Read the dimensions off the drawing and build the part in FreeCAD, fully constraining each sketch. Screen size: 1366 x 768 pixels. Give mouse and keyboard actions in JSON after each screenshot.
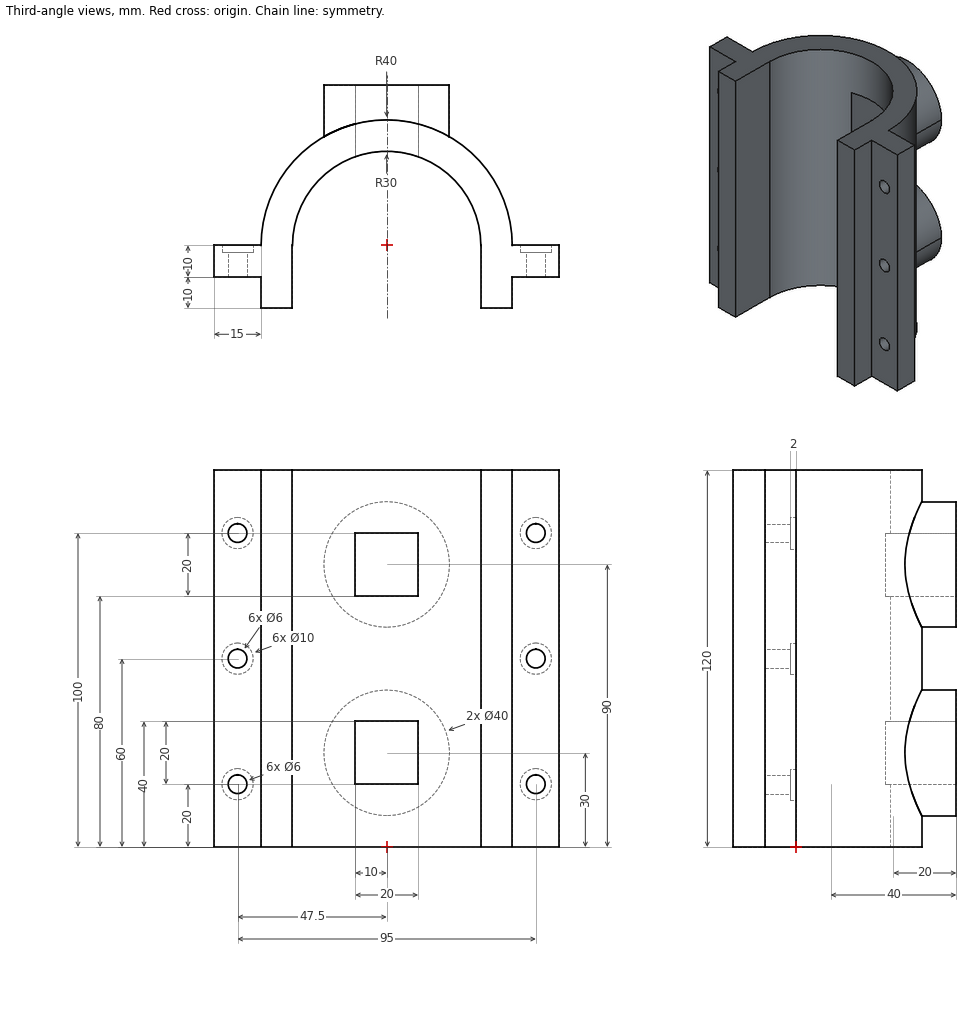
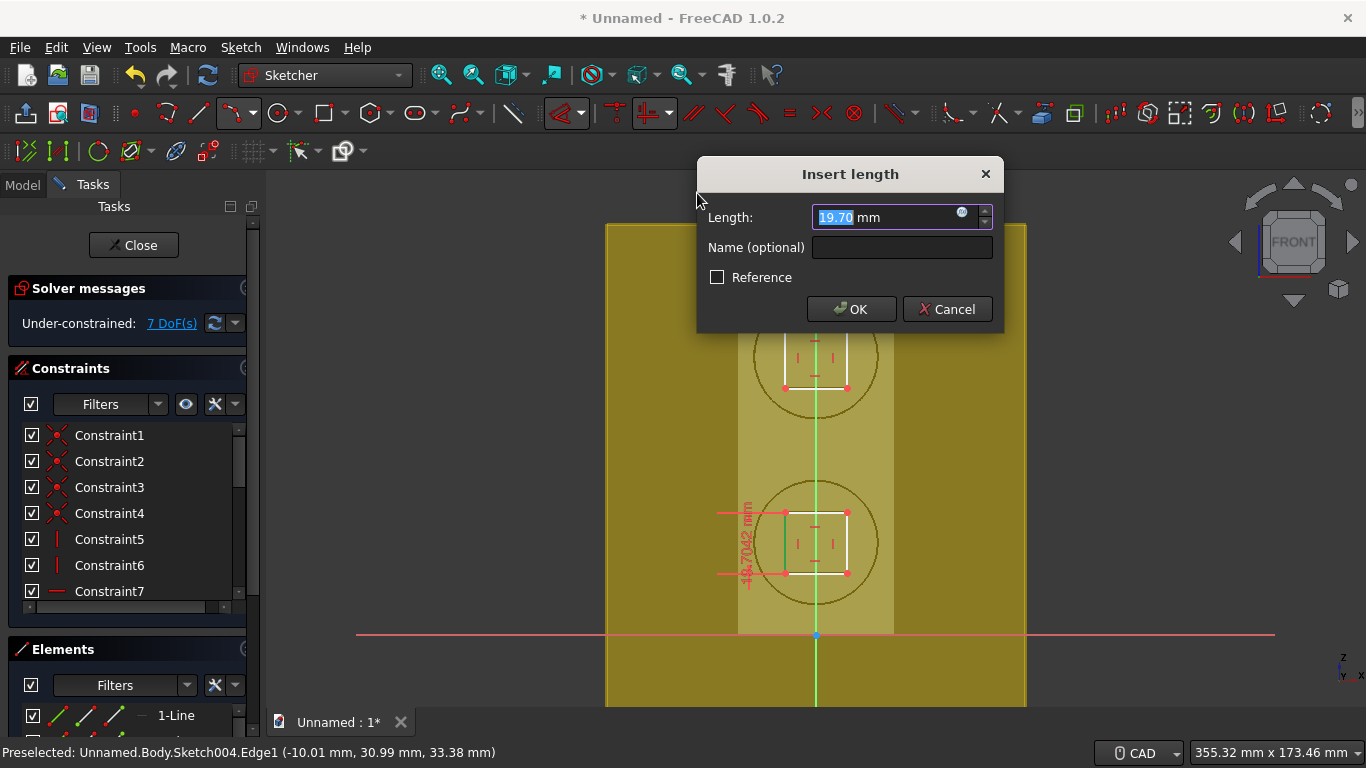
{"action": "type", "text": "20"}
{"action": "key", "text": "Return"}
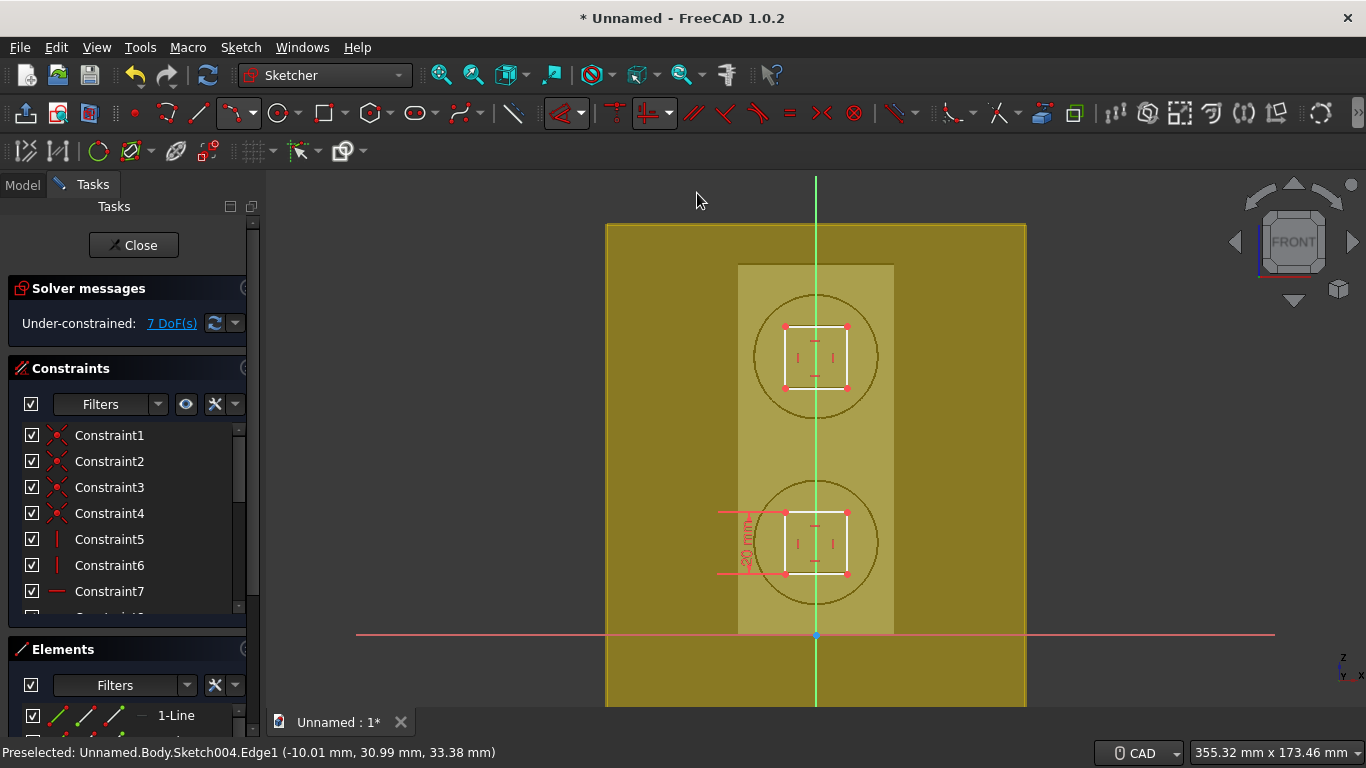
{"action": "left_click", "coordinate": [804, 574]}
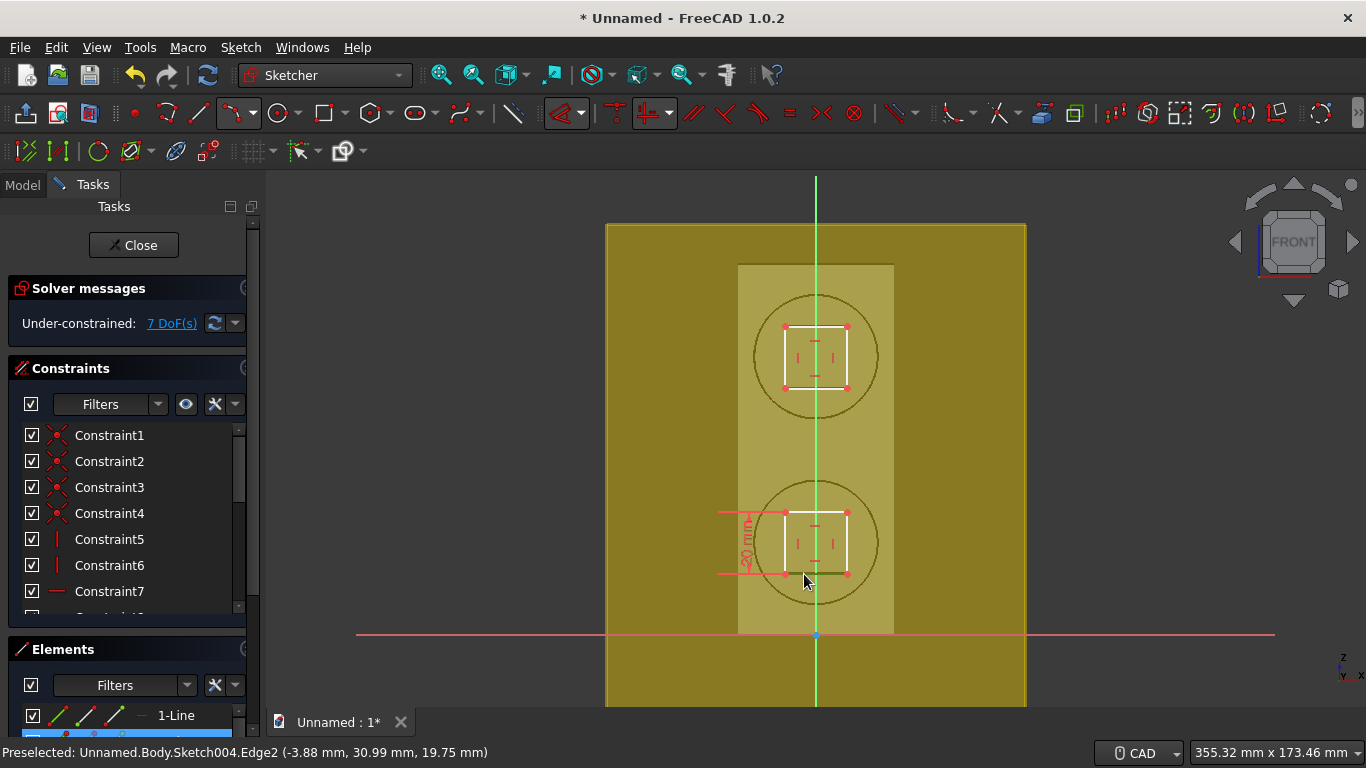
{"action": "key", "text": "l"}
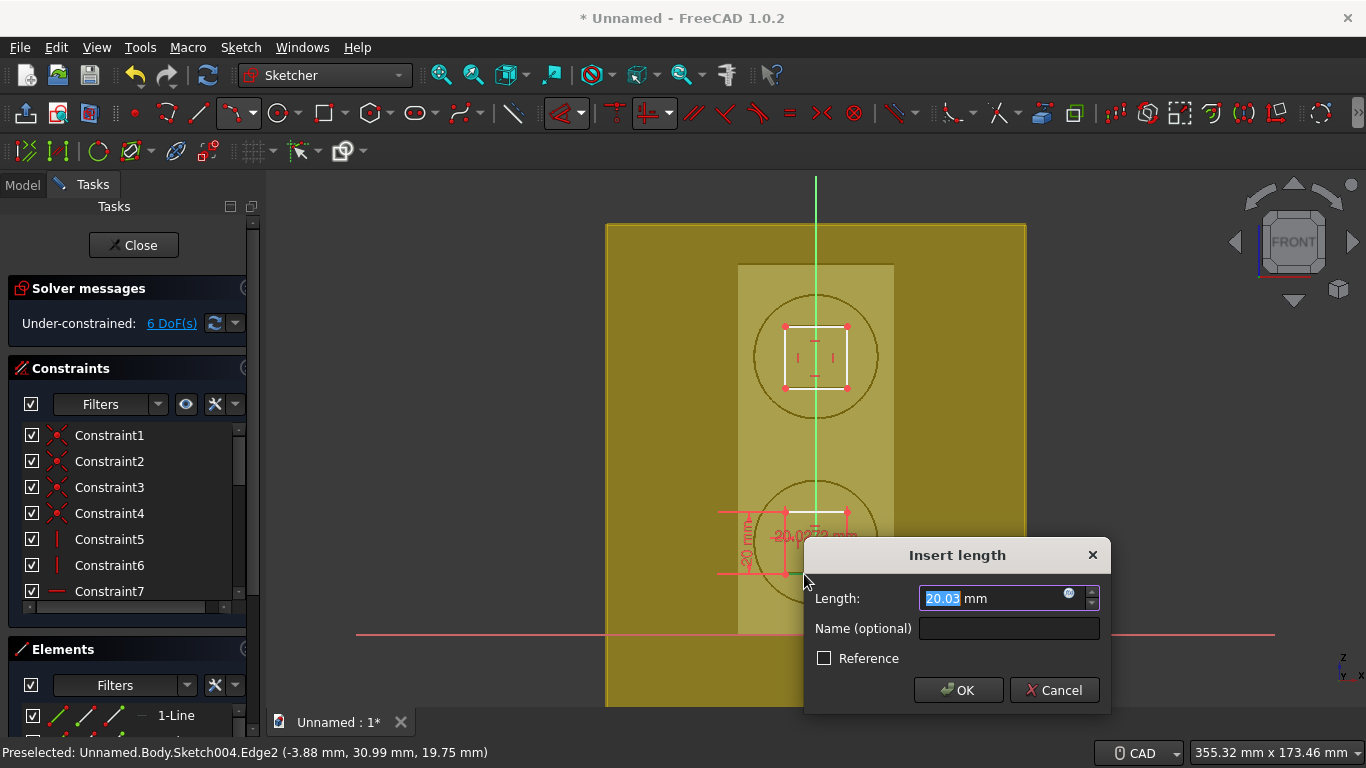
{"action": "type", "text": "20"}
{"action": "key", "text": "Return"}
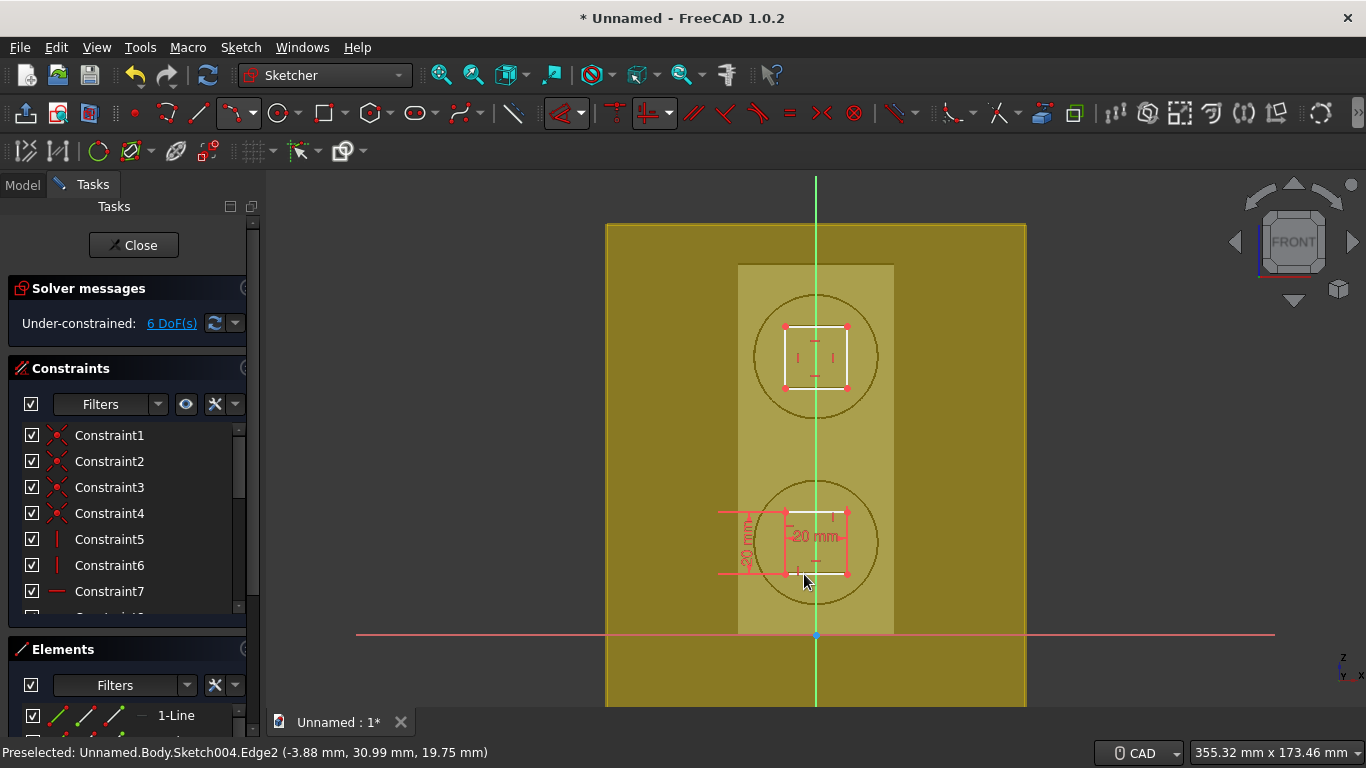
{"action": "left_click", "coordinate": [785, 346]}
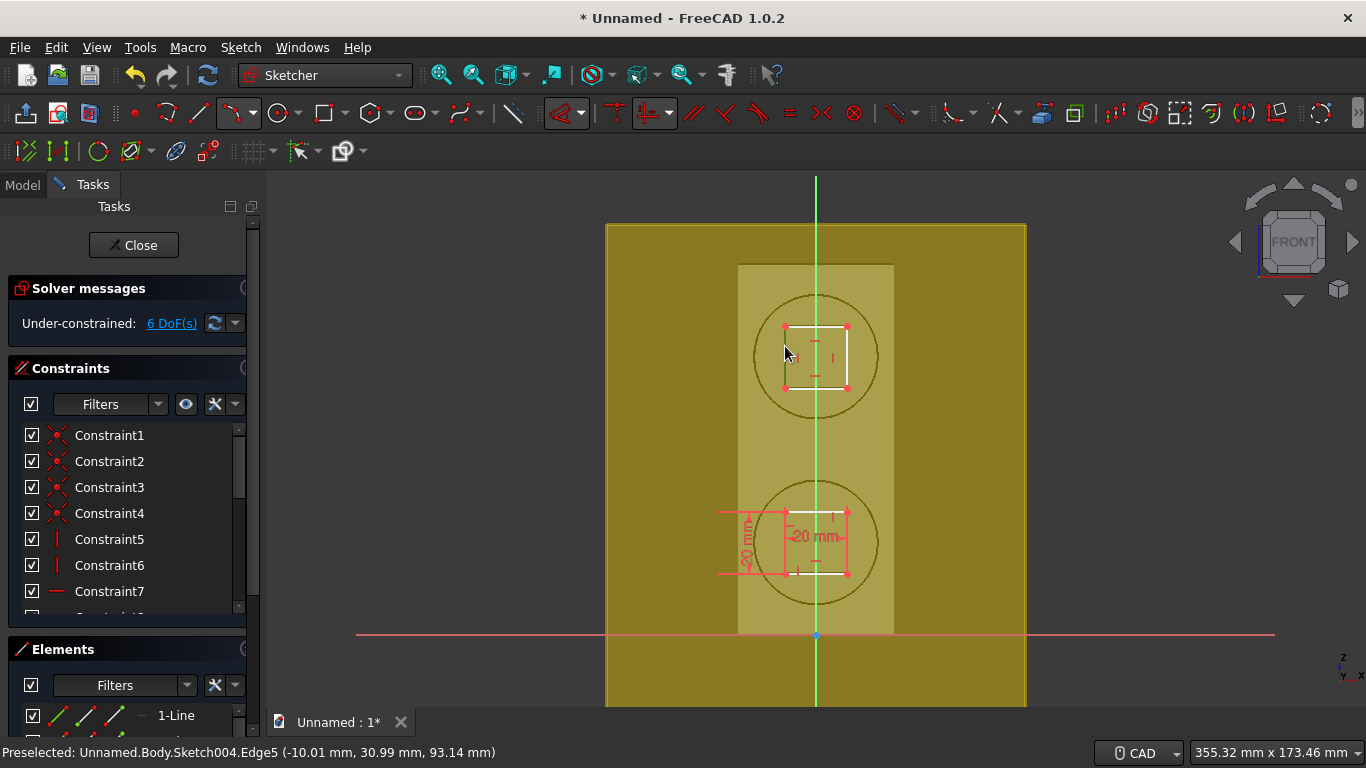
{"action": "left_click", "coordinate": [584, 114]}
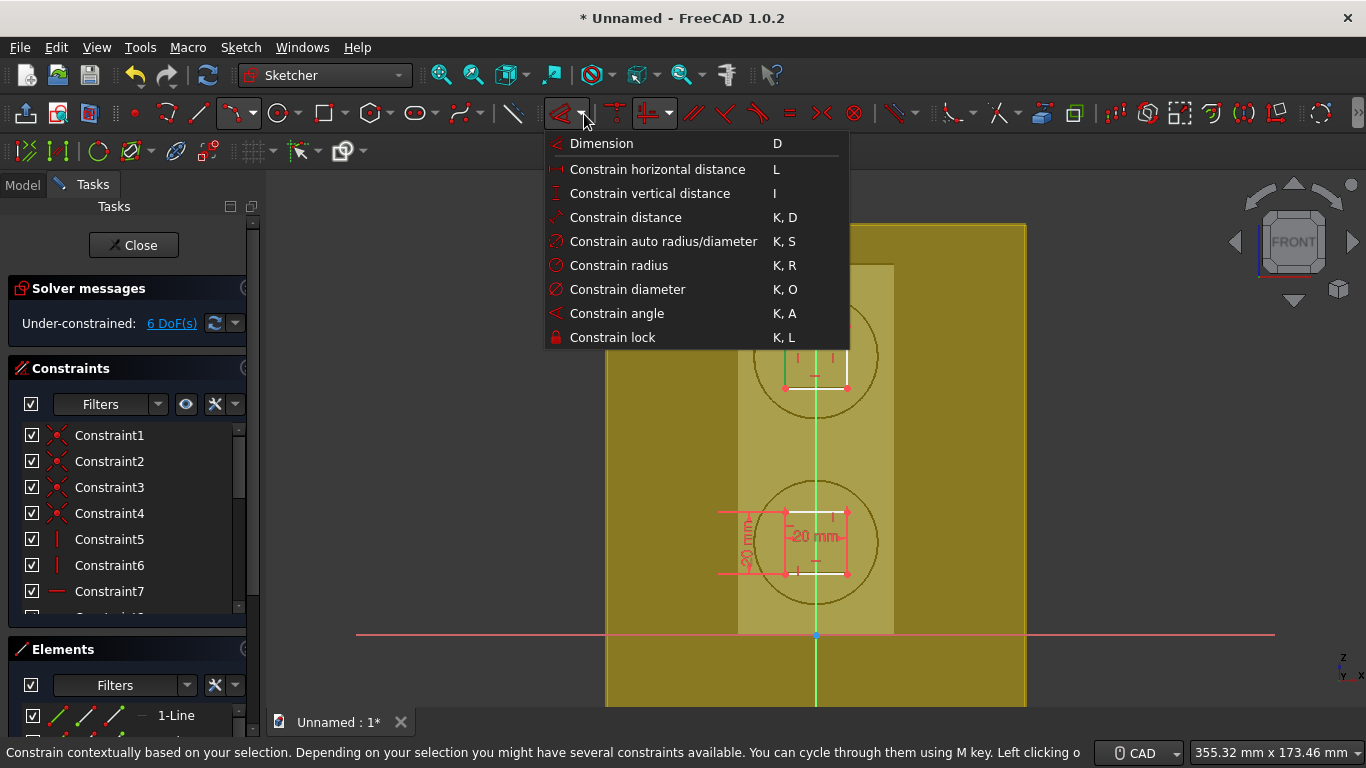
{"action": "left_click", "coordinate": [697, 193]}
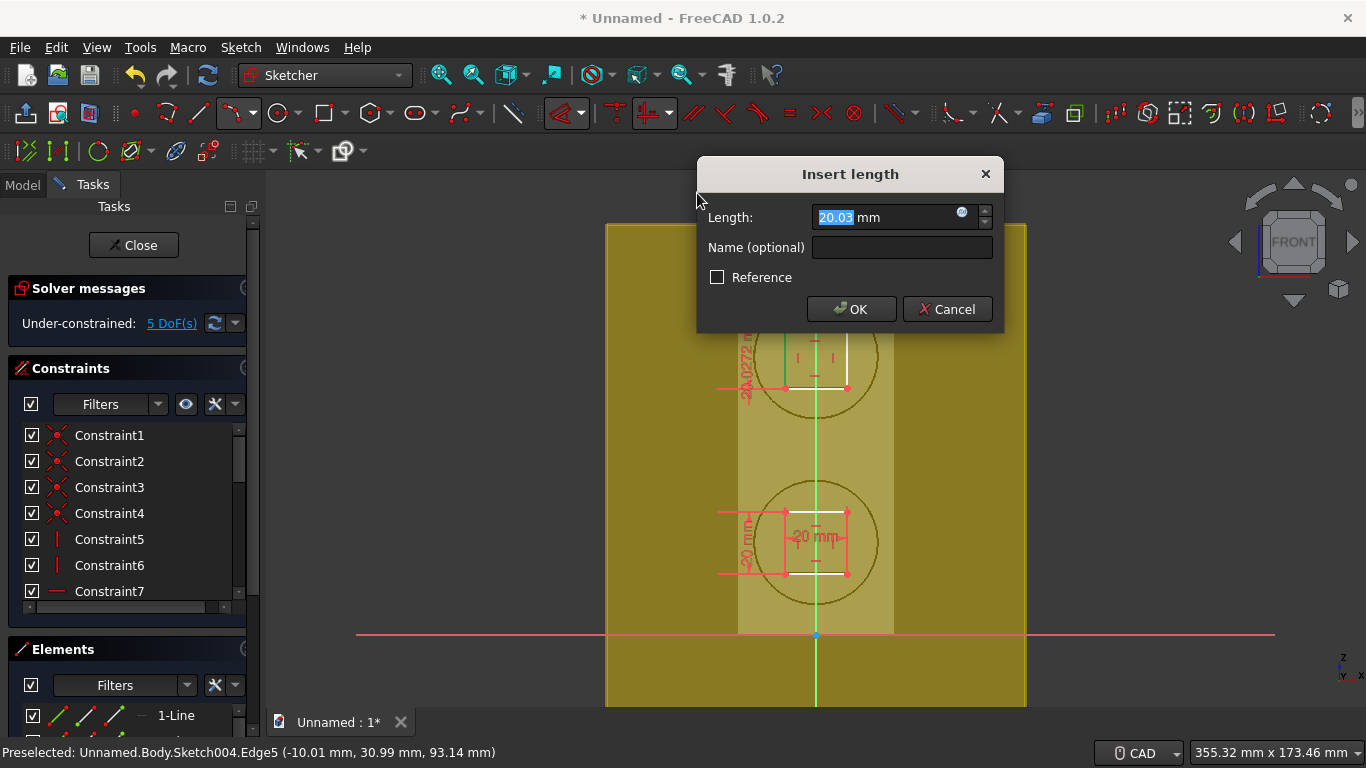
{"action": "type", "text": "20"}
{"action": "key", "text": "Return"}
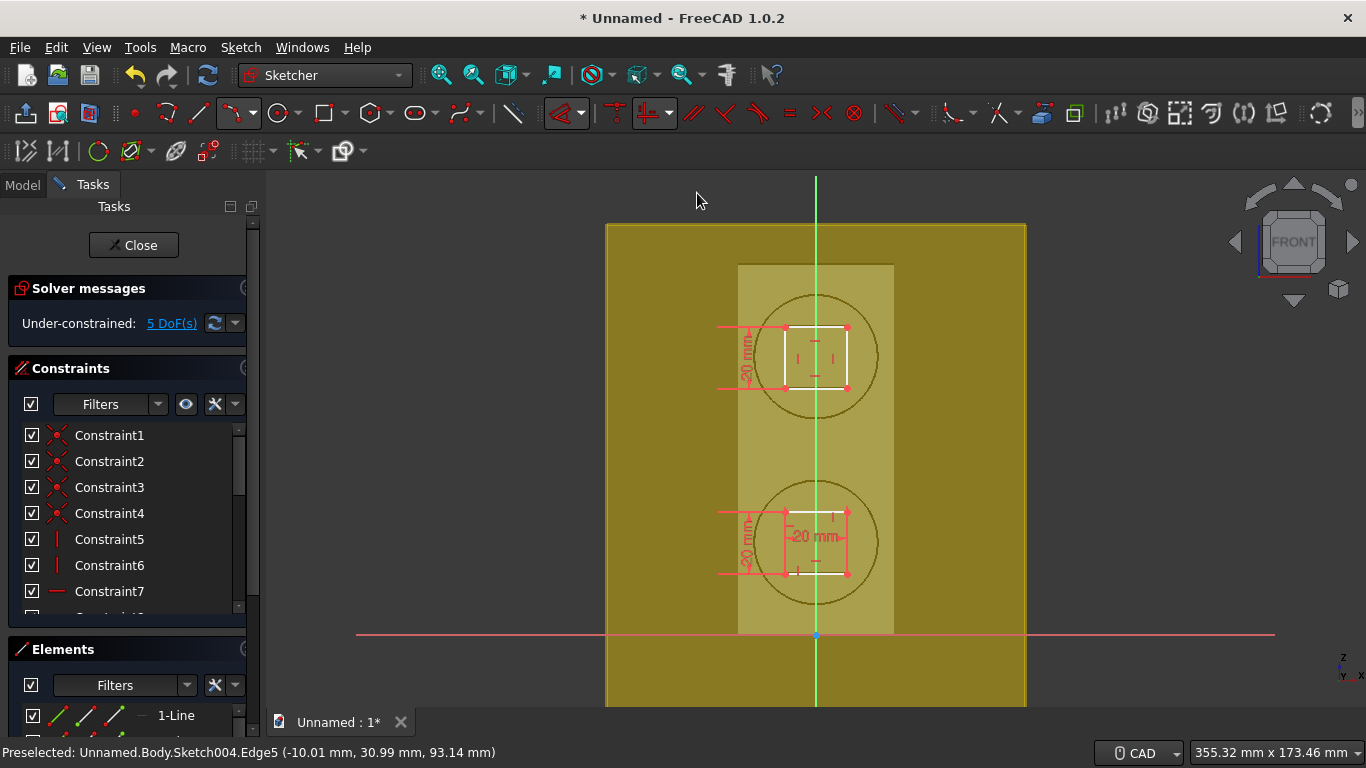
{"action": "left_click", "coordinate": [804, 389]}